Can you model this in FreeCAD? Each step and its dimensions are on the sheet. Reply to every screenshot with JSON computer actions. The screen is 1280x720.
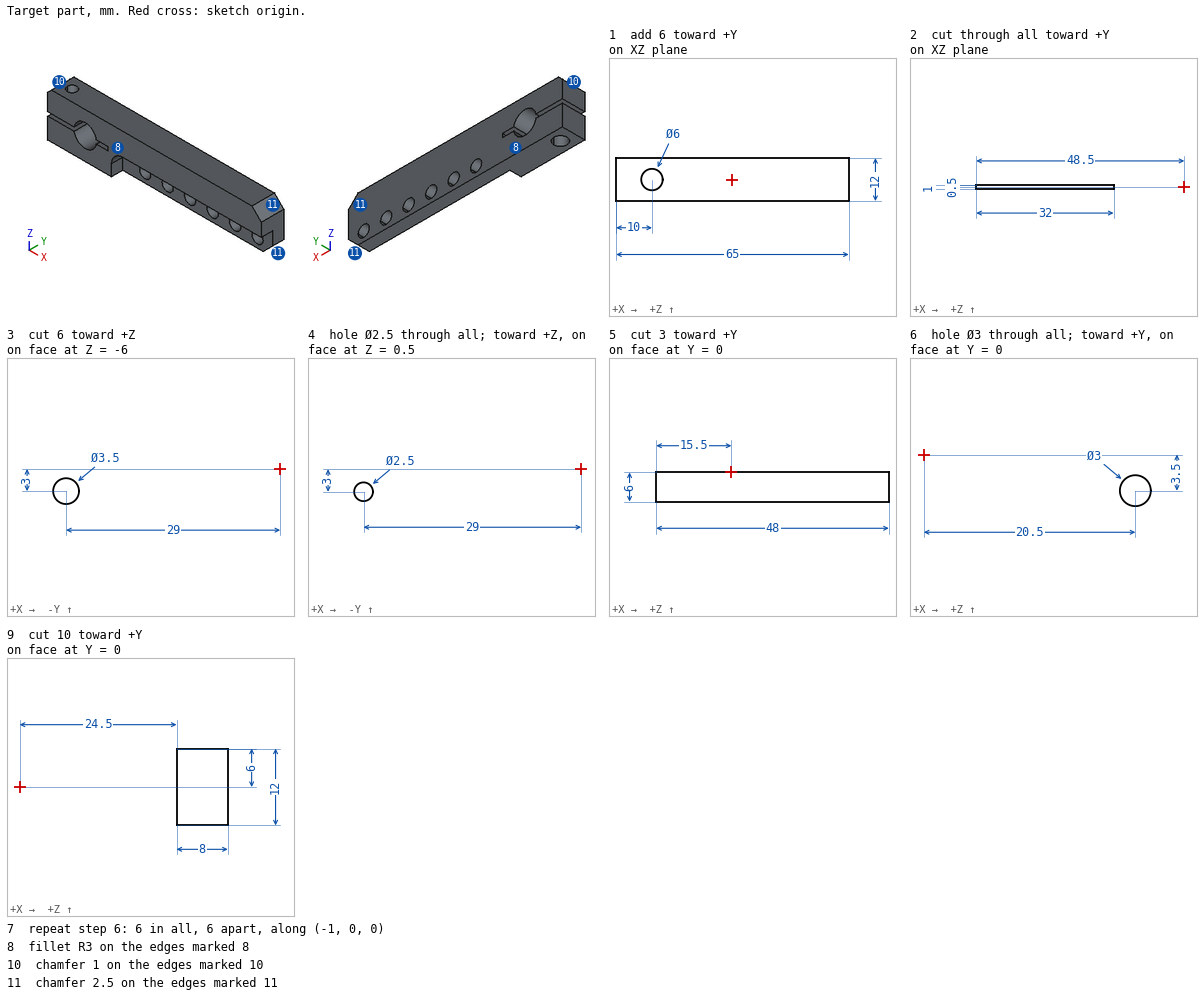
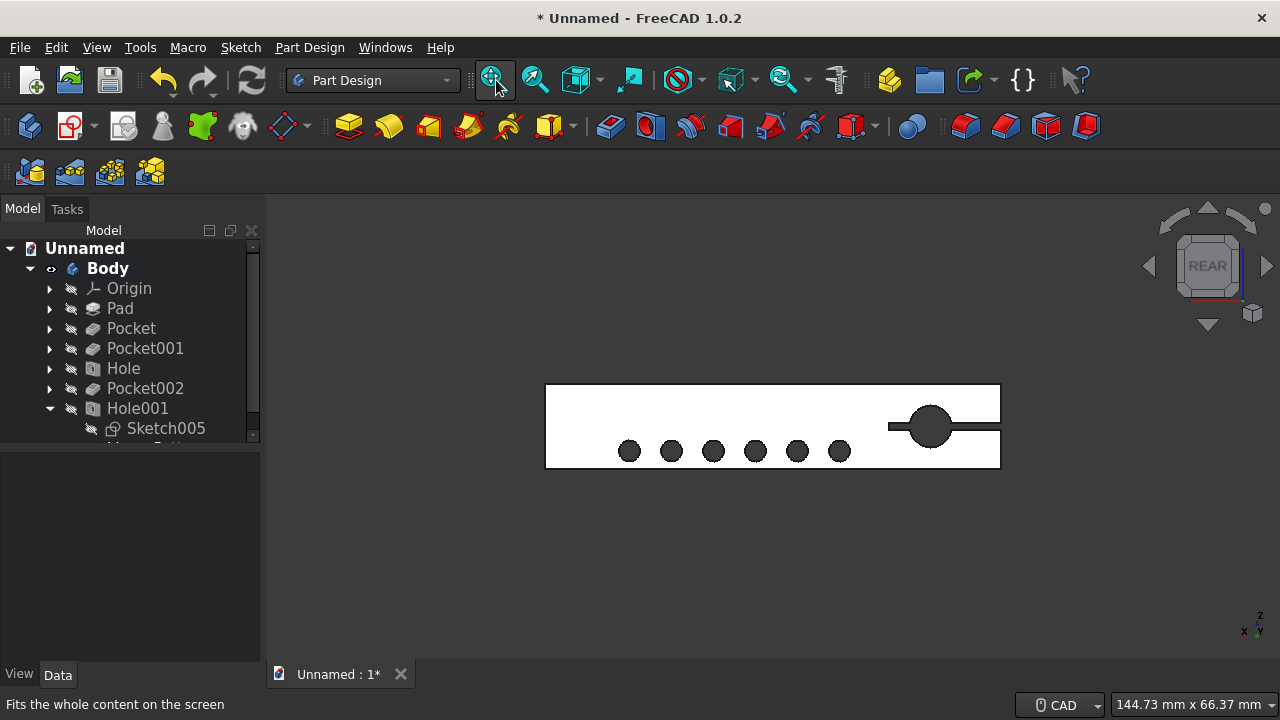
{"action": "key", "text": "6"}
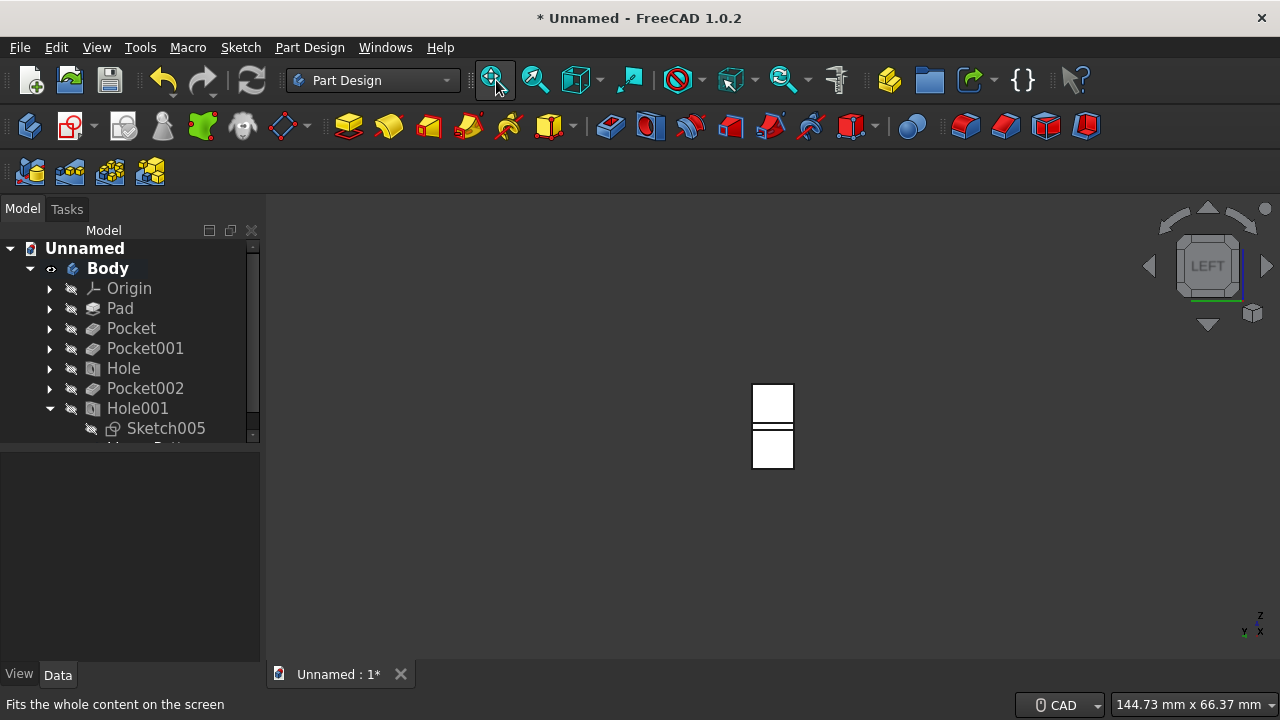
{"action": "left_click", "coordinate": [496, 80]}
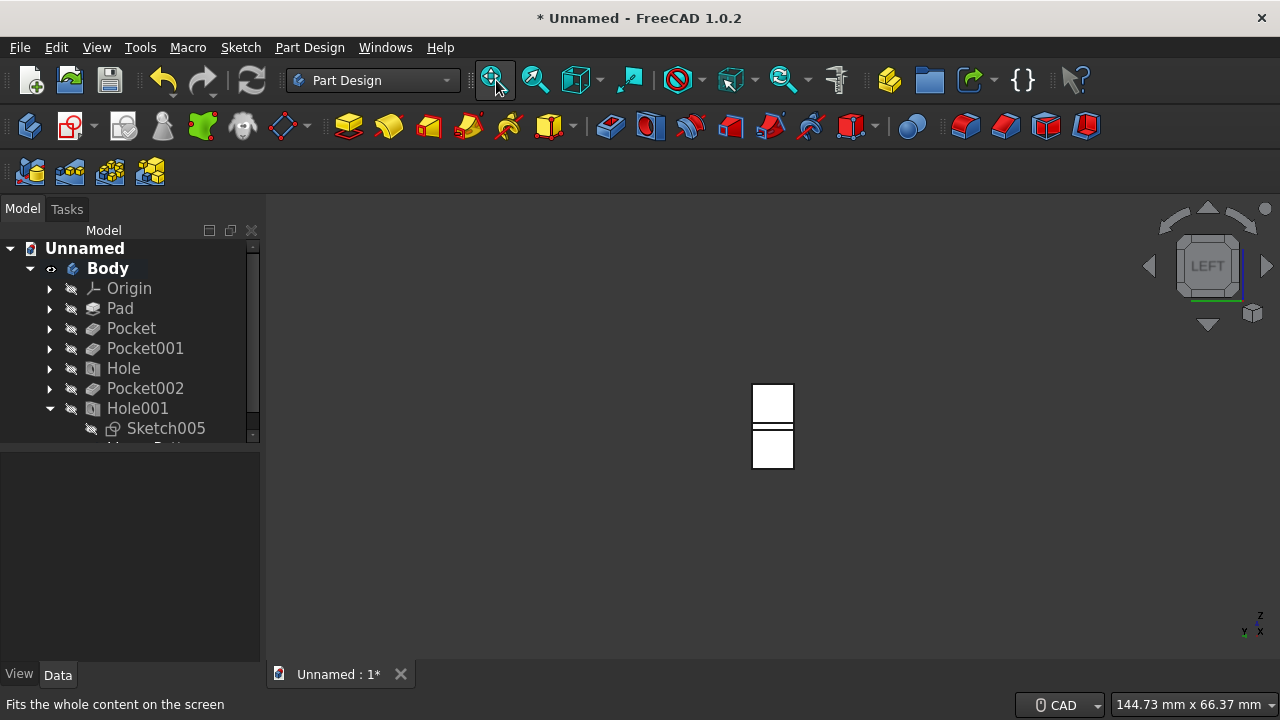
{"action": "scroll", "coordinate": [784, 425], "scroll_direction": "up", "scroll_amount": 4}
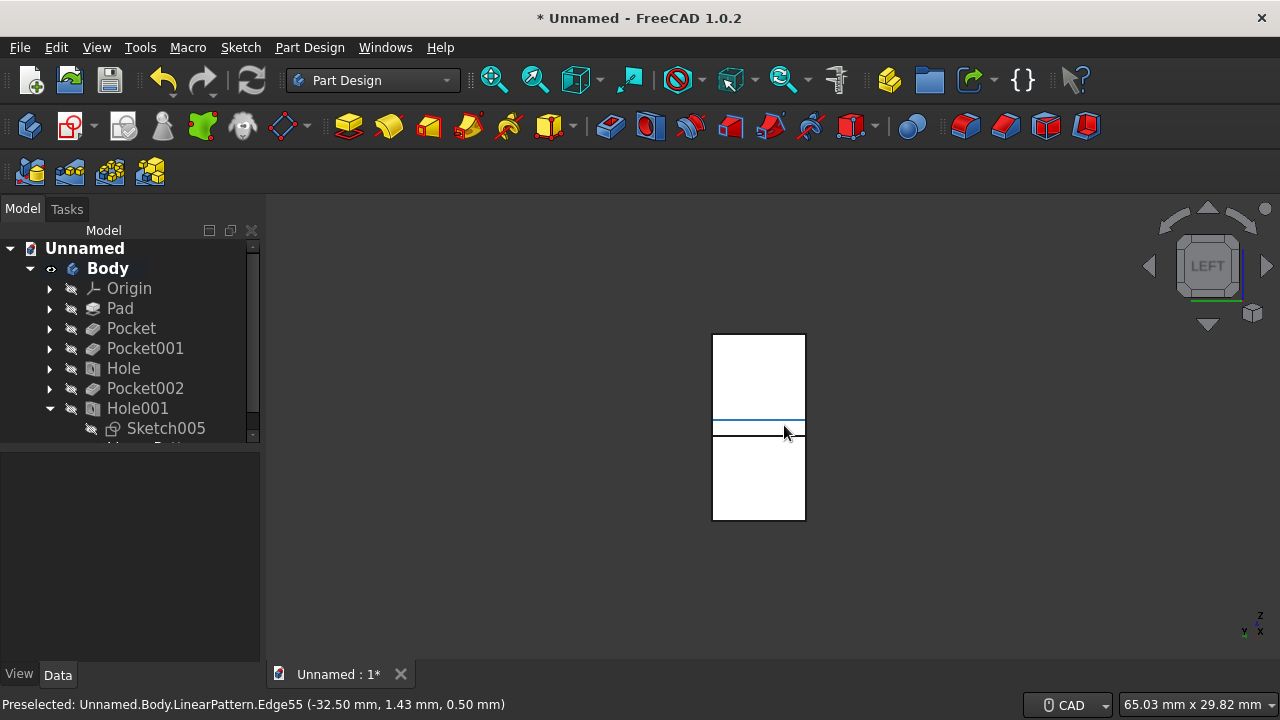
{"action": "key", "text": "v f"}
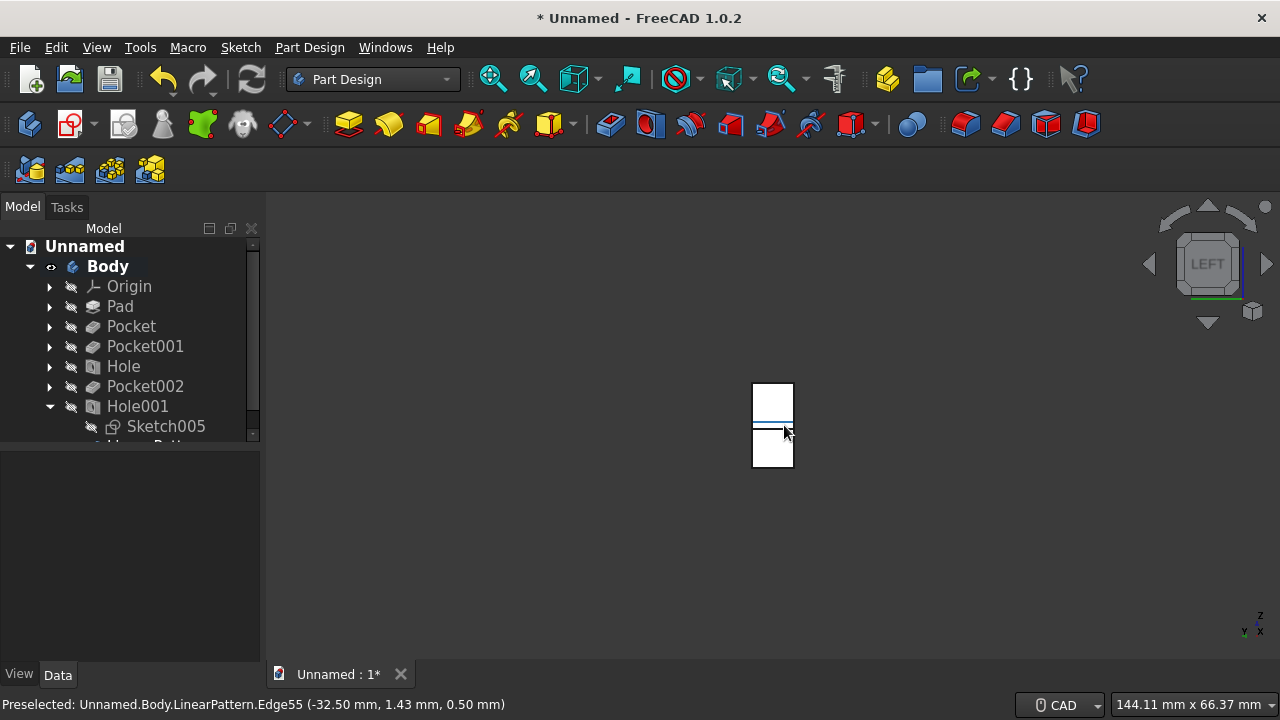
{"action": "key", "text": "v 3"}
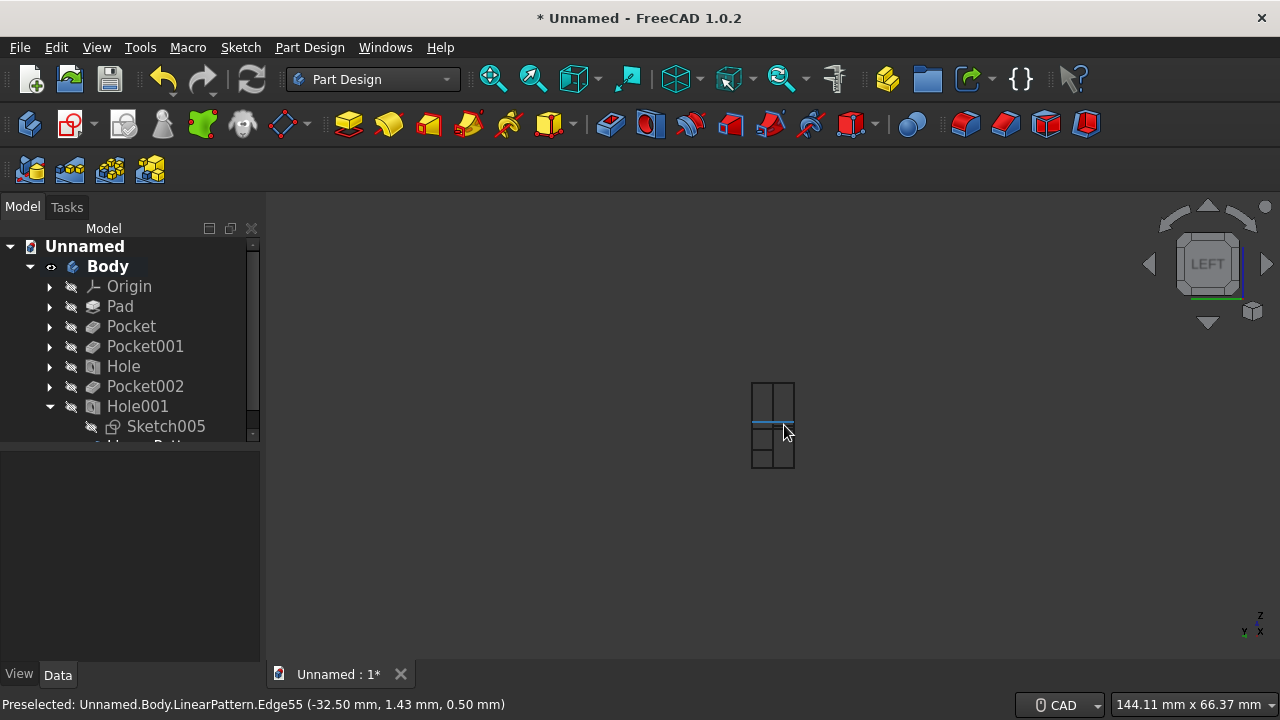
{"action": "key", "text": "0"}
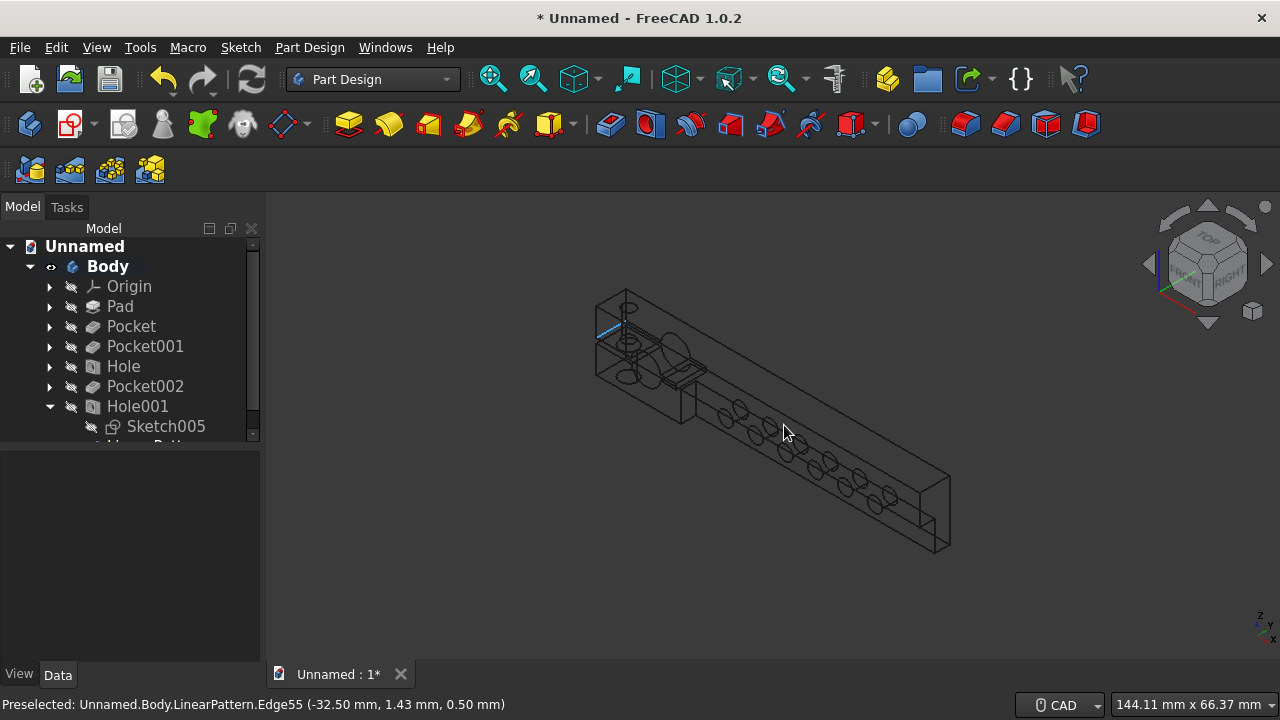
{"action": "left_click", "coordinate": [688, 384]}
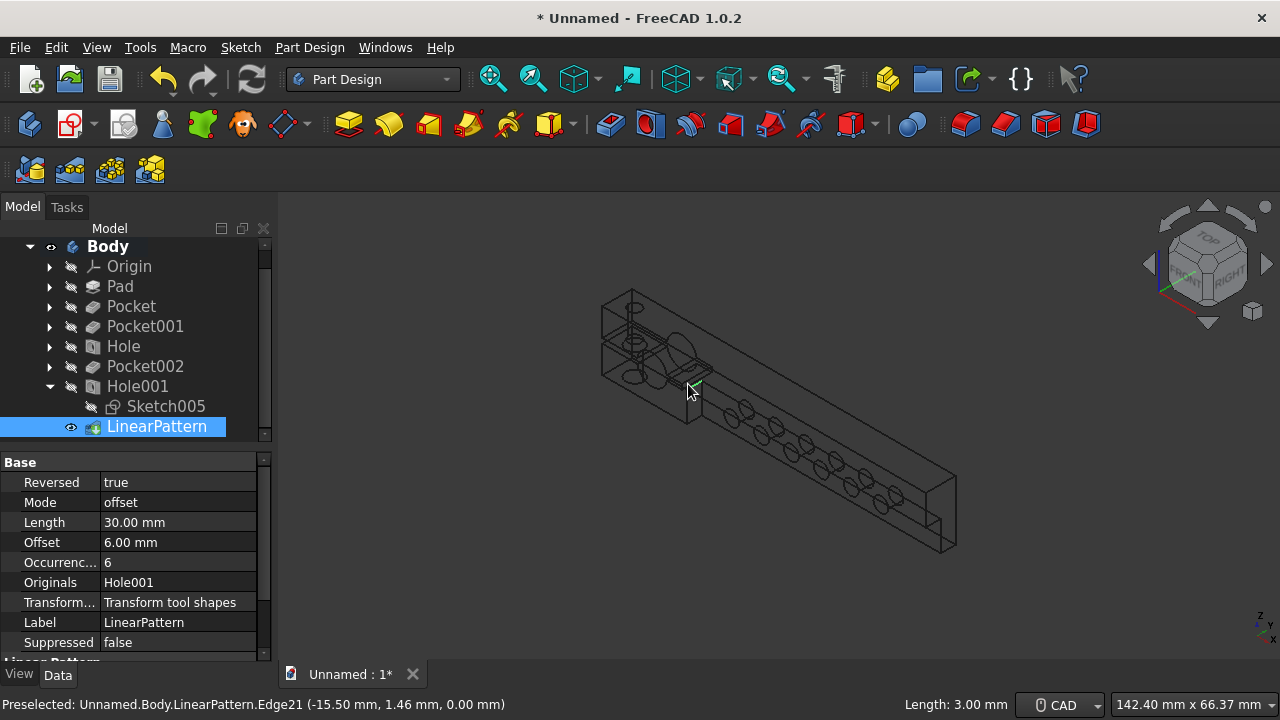
{"action": "key", "text": "v 1"}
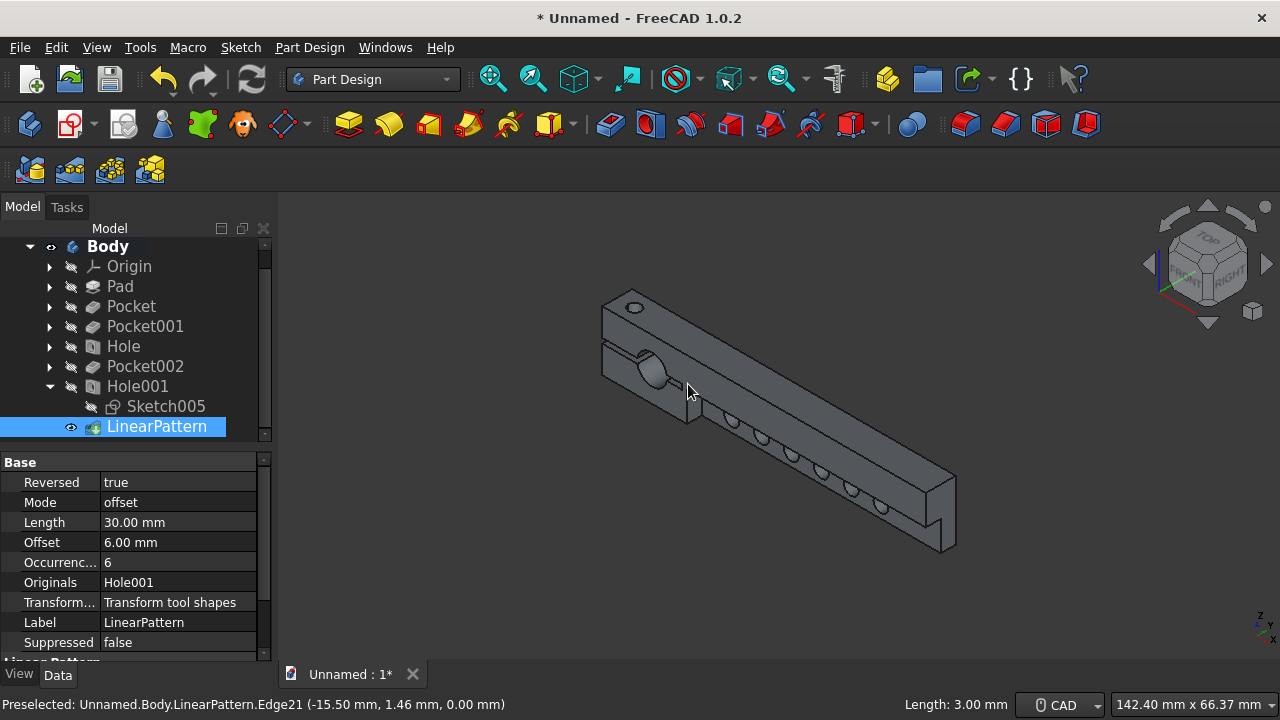
{"action": "left_click", "coordinate": [966, 124]}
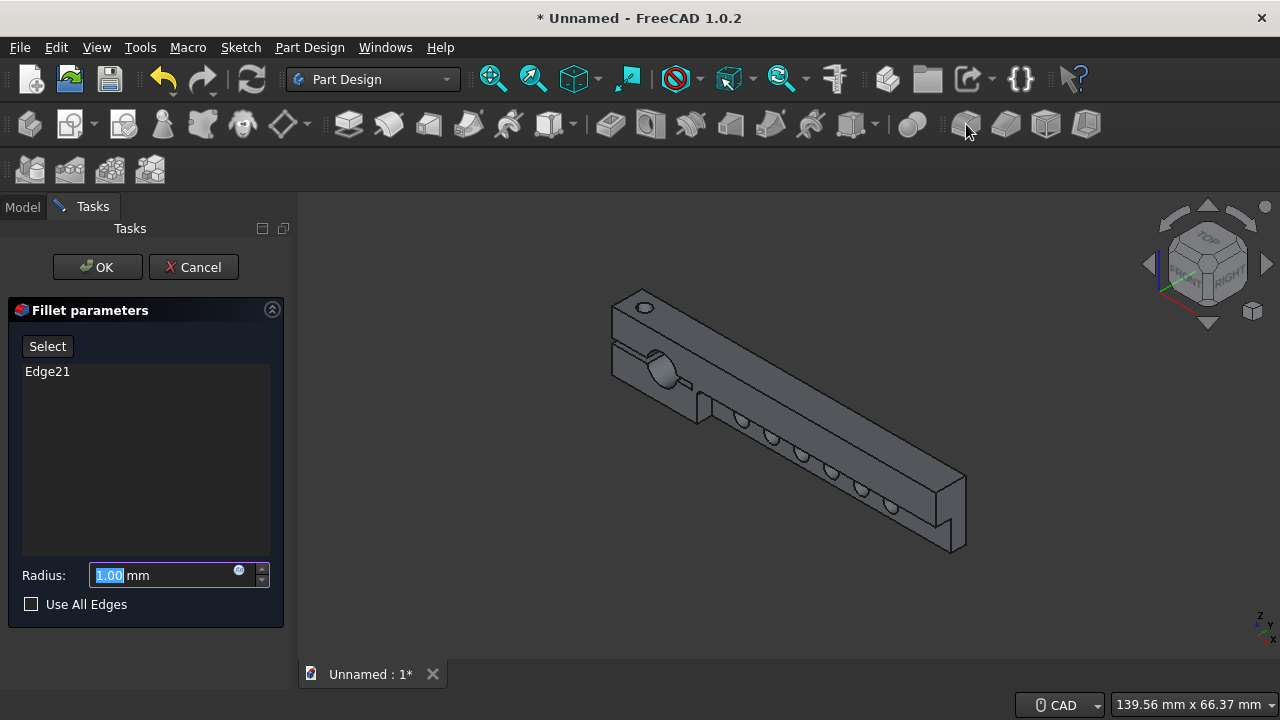
{"action": "type", "text": "3"}
{"action": "key", "text": "Tab"}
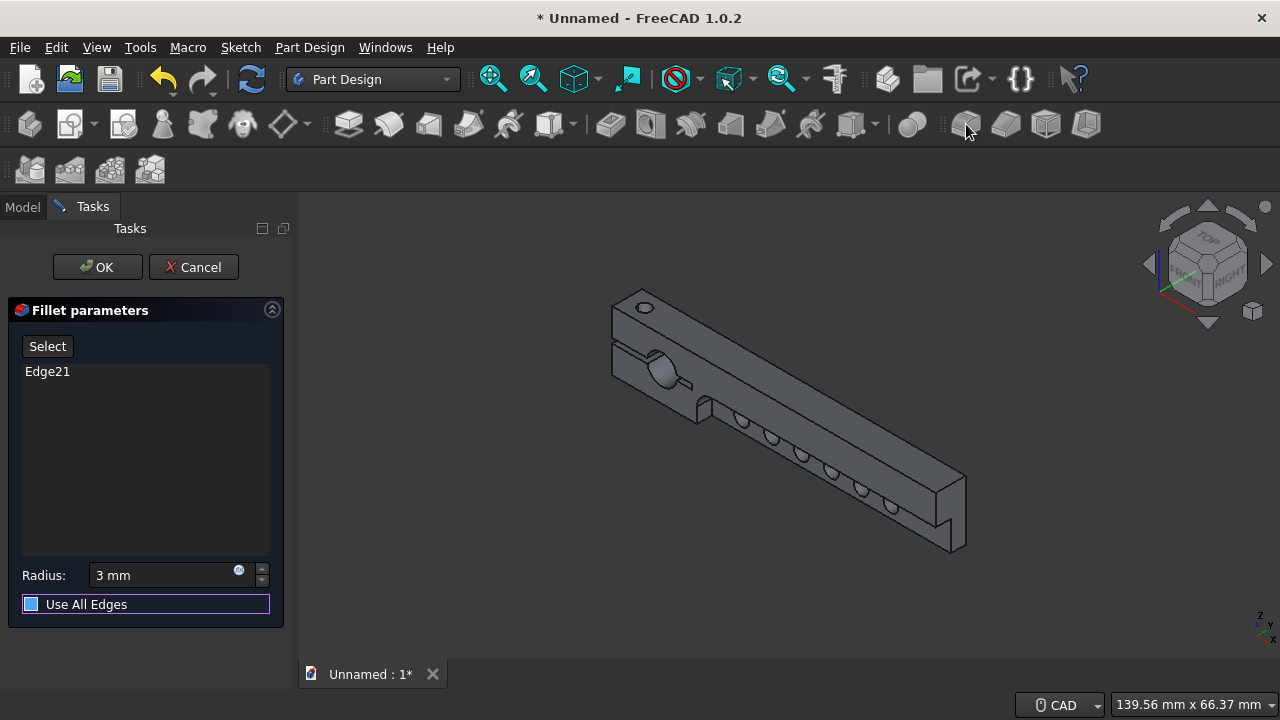
{"action": "left_click", "coordinate": [98, 267]}